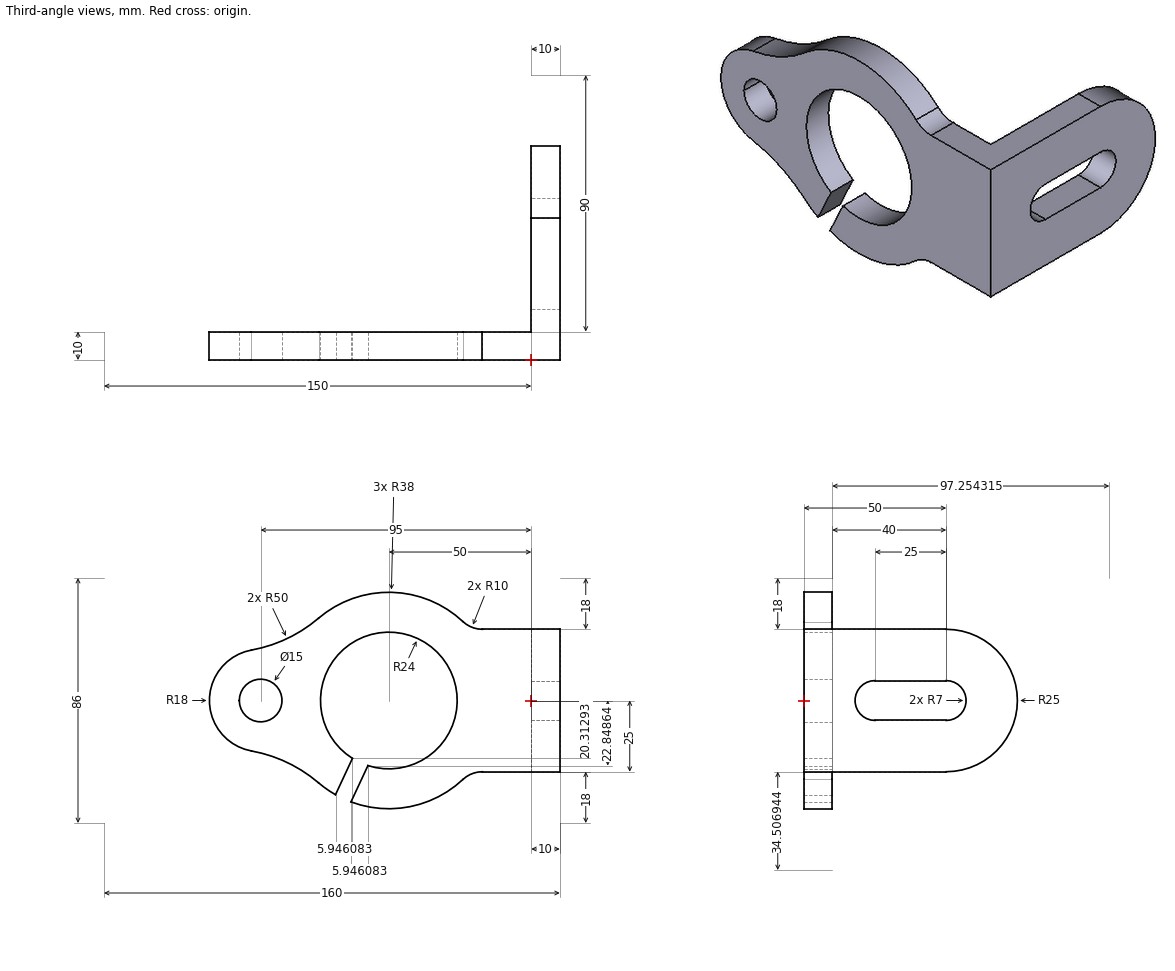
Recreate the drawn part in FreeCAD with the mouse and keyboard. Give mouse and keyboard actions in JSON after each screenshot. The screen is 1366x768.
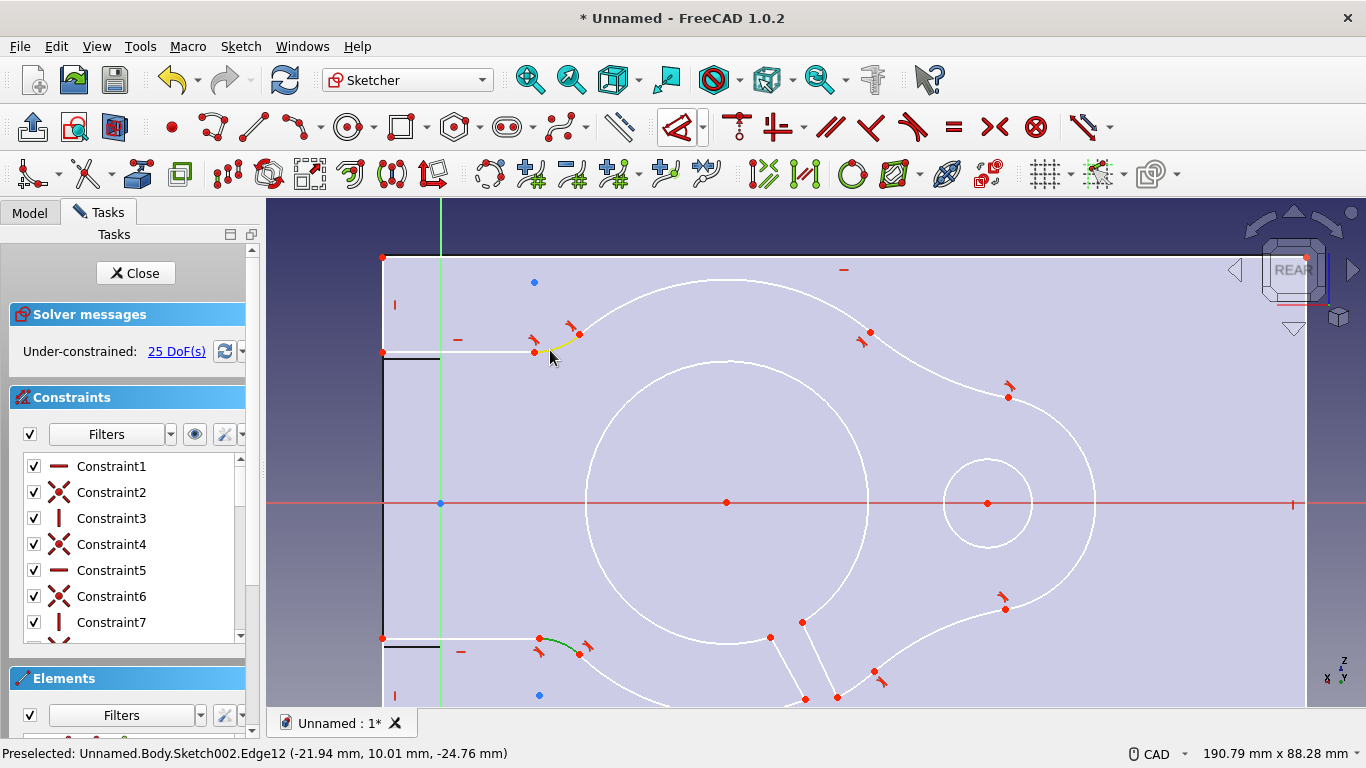
{"action": "left_click", "coordinate": [549, 350]}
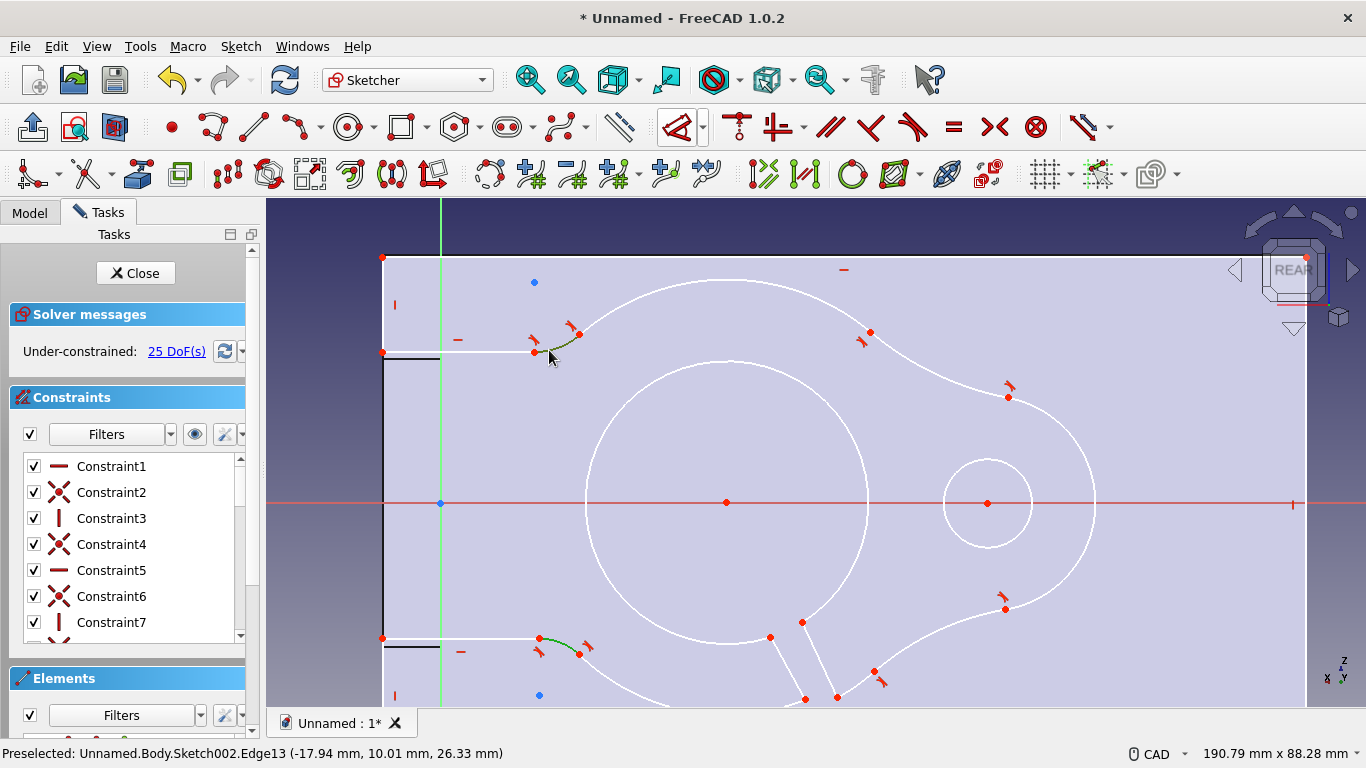
{"action": "key", "text": "e"}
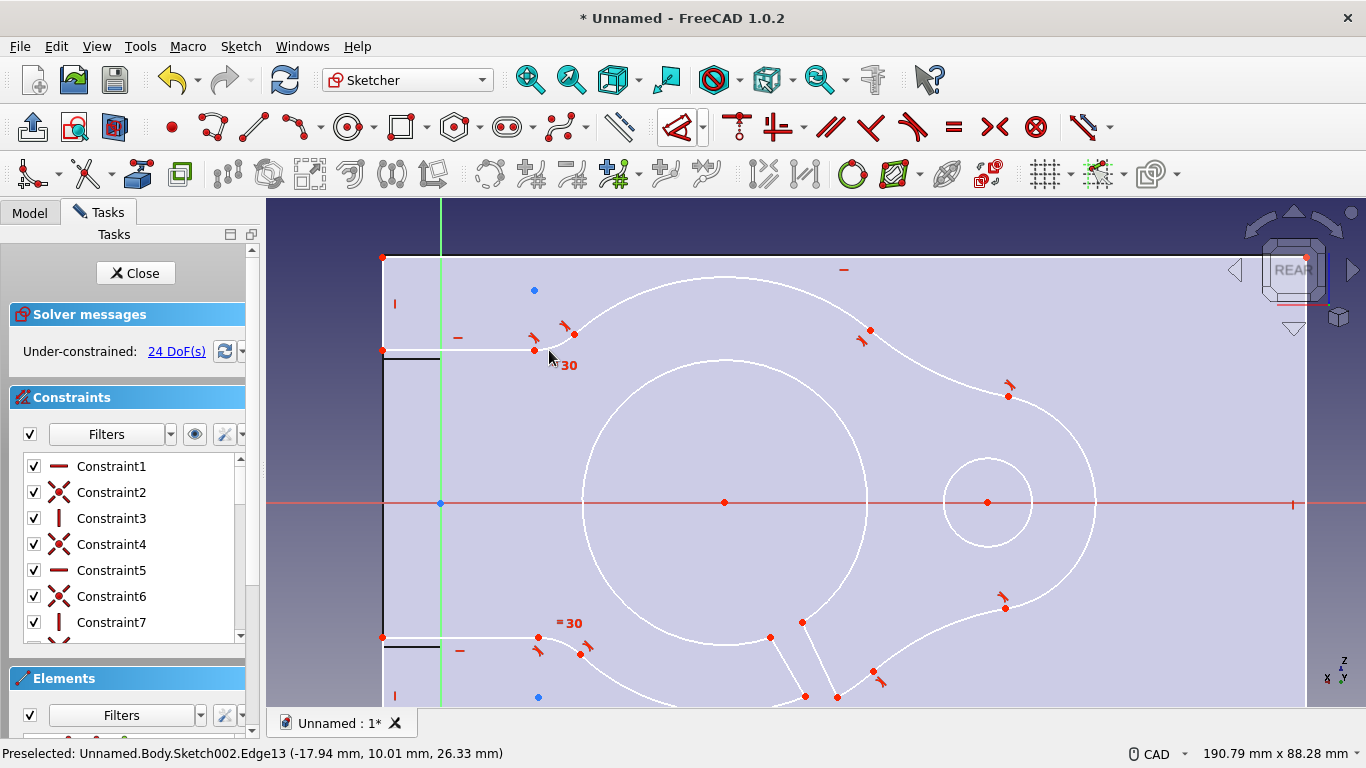
{"action": "scroll", "coordinate": [550, 349], "scroll_direction": "down", "scroll_amount": 2}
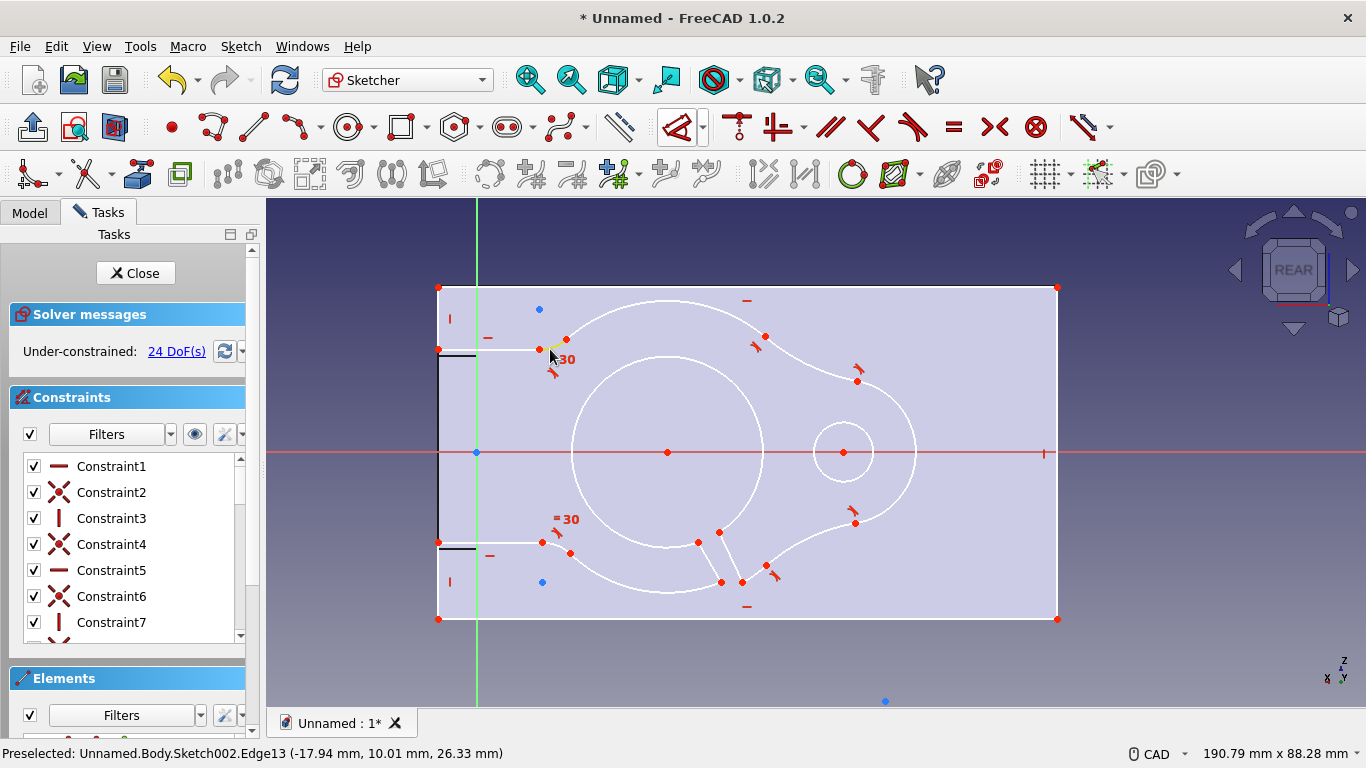
{"action": "left_click", "coordinate": [611, 581]}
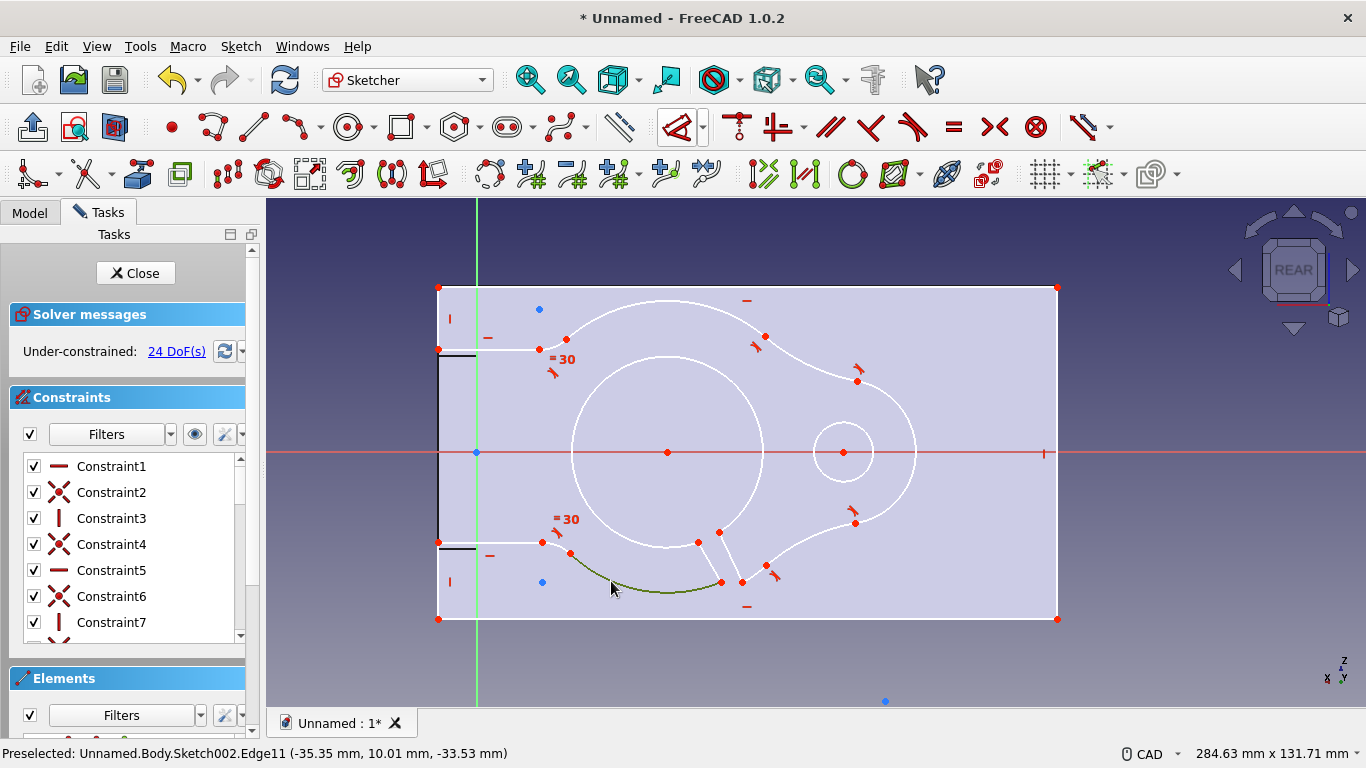
{"action": "left_click", "coordinate": [708, 307]}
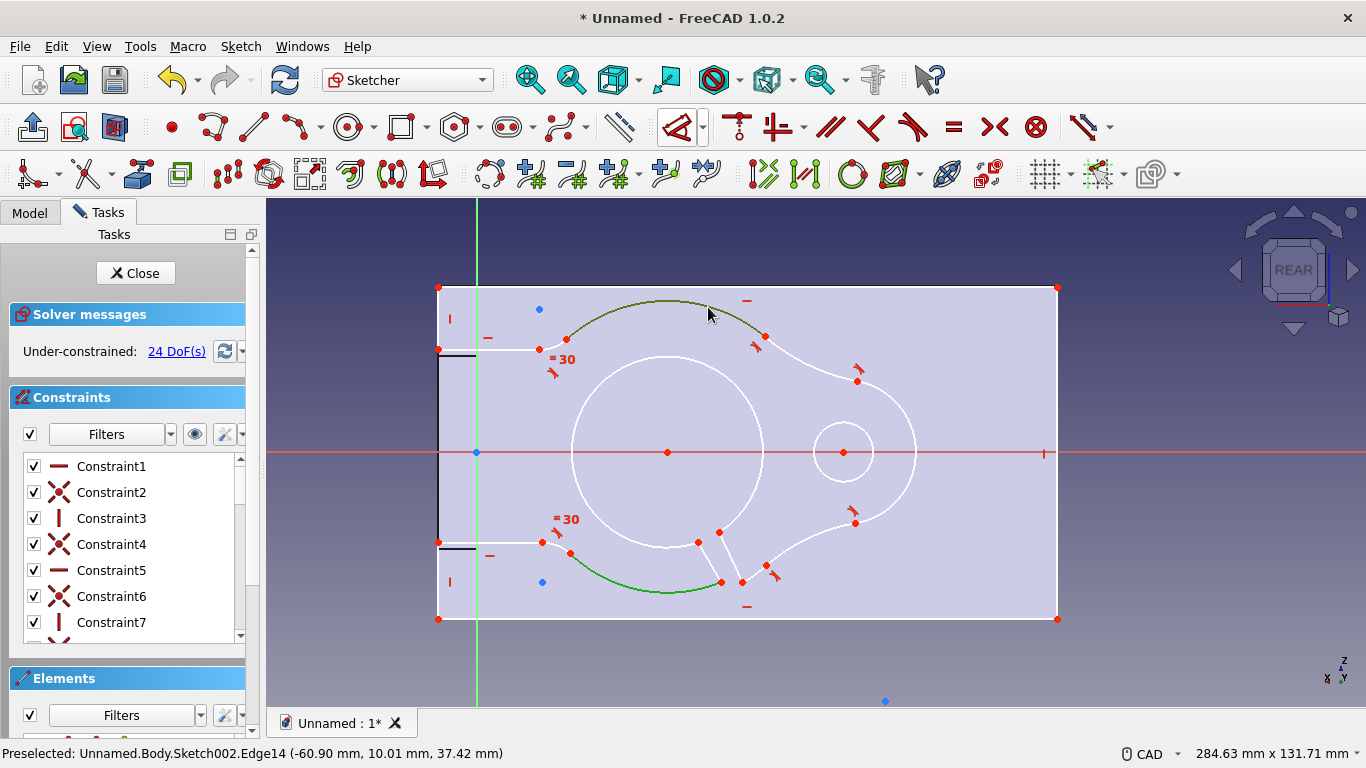
{"action": "left_click", "coordinate": [755, 575]}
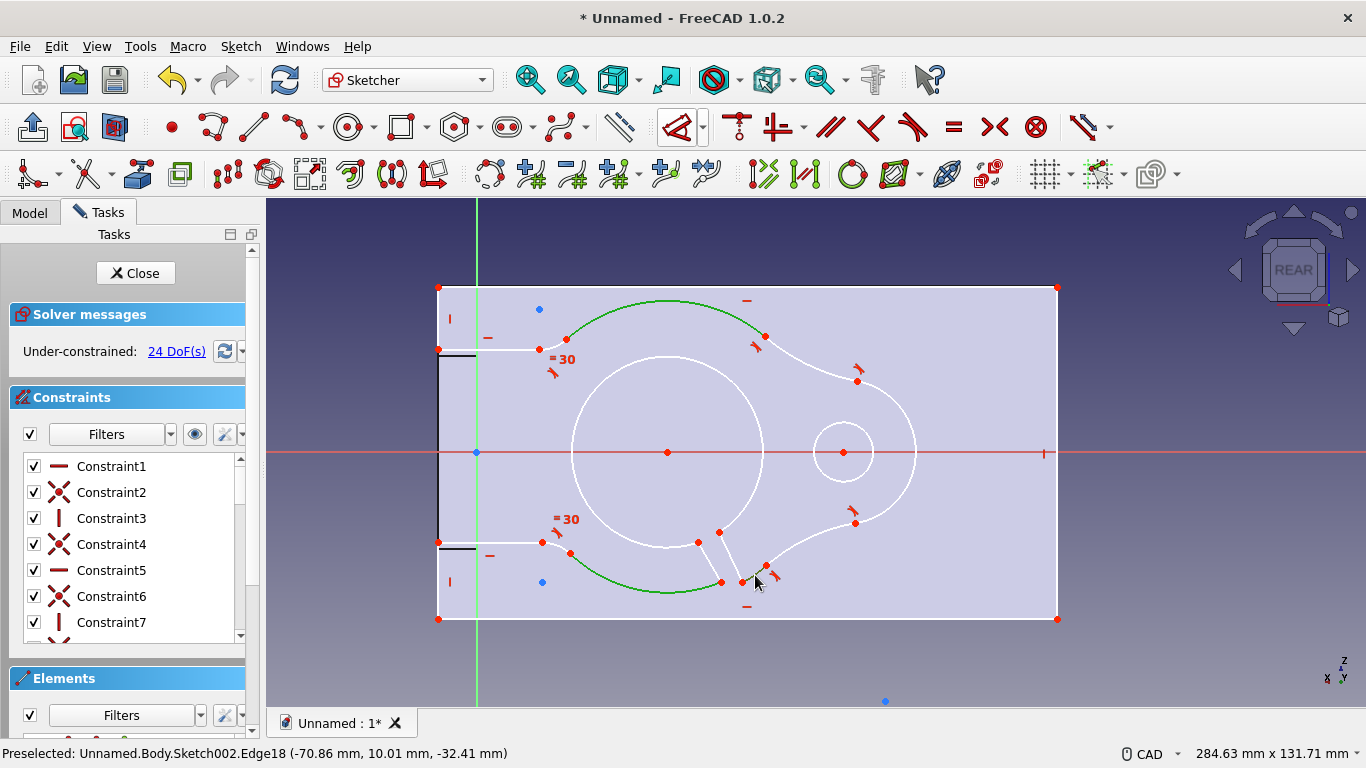
{"action": "key", "text": "e"}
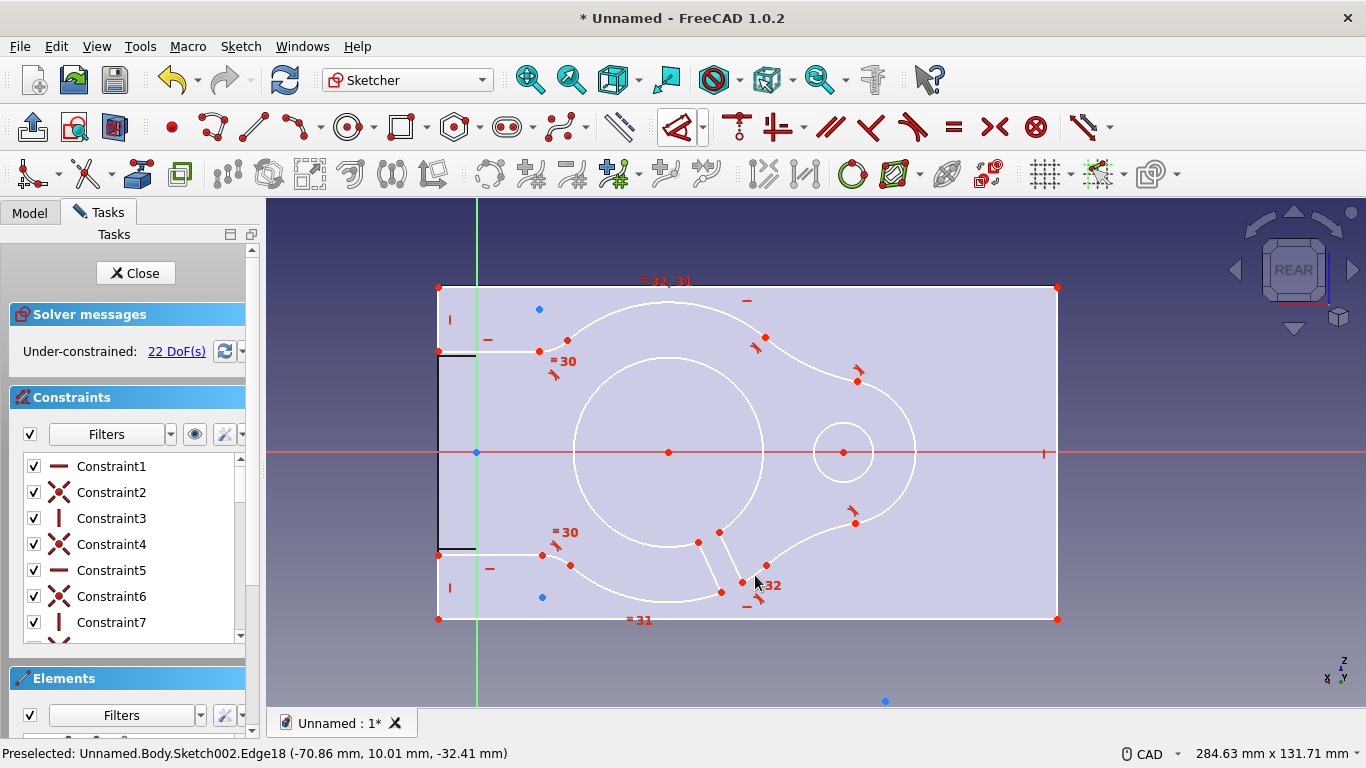
{"action": "left_click", "coordinate": [790, 356]}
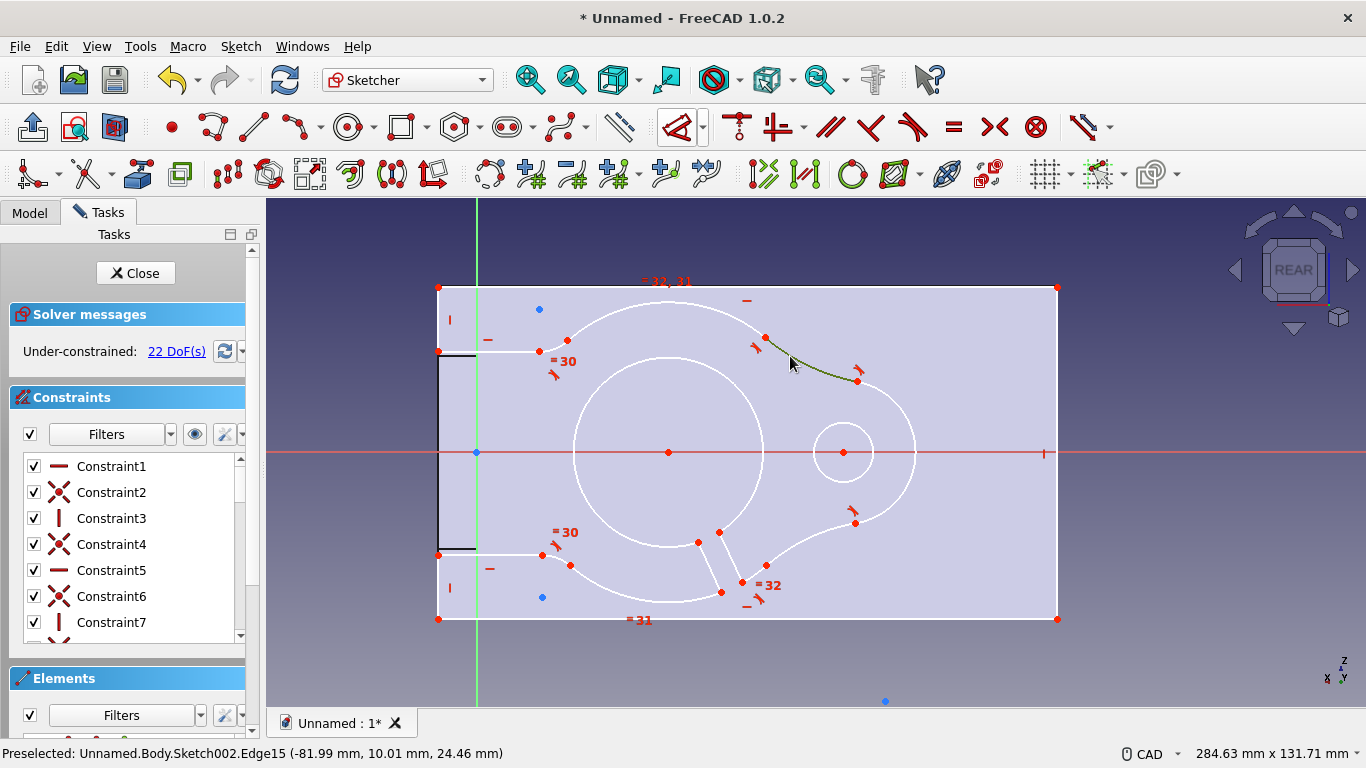
{"action": "left_click", "coordinate": [827, 531]}